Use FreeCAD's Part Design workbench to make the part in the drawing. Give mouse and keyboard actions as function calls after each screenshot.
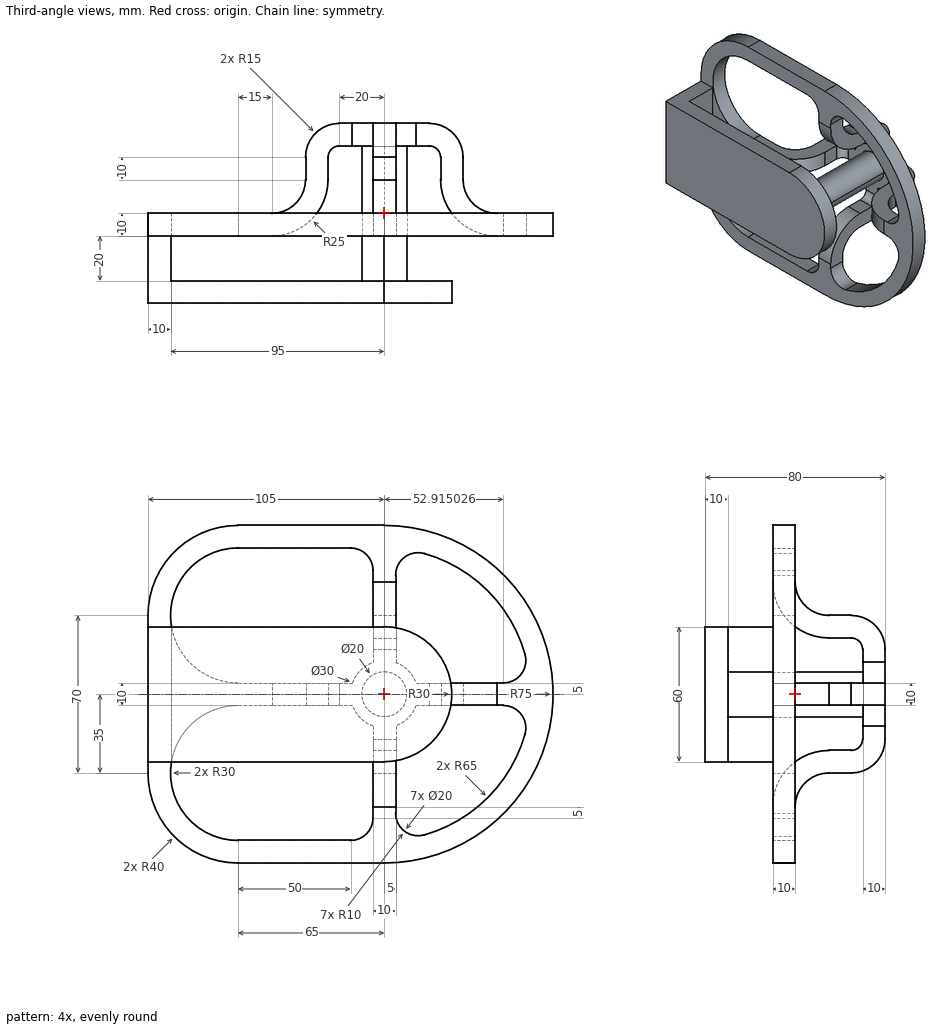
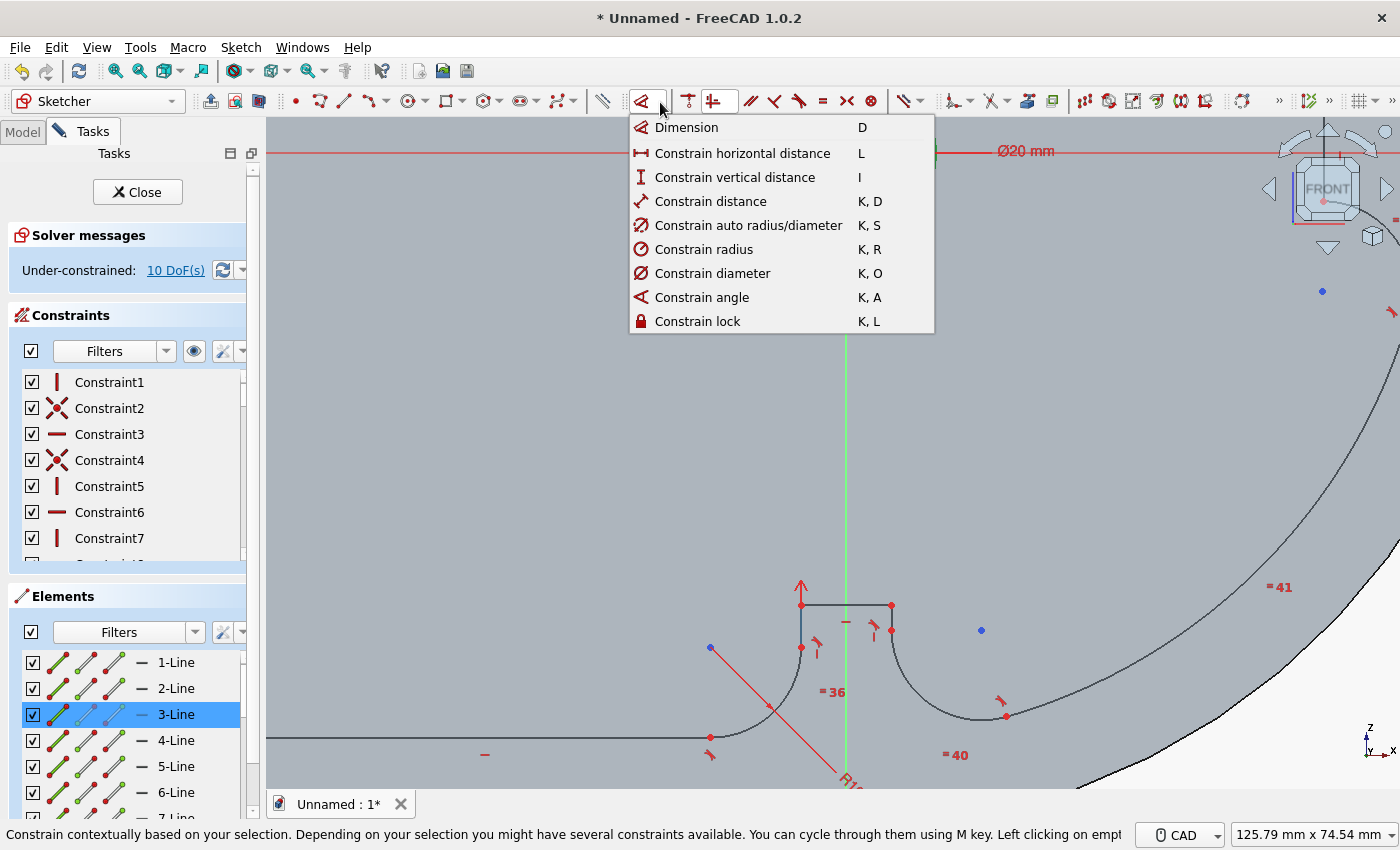
click(782, 177)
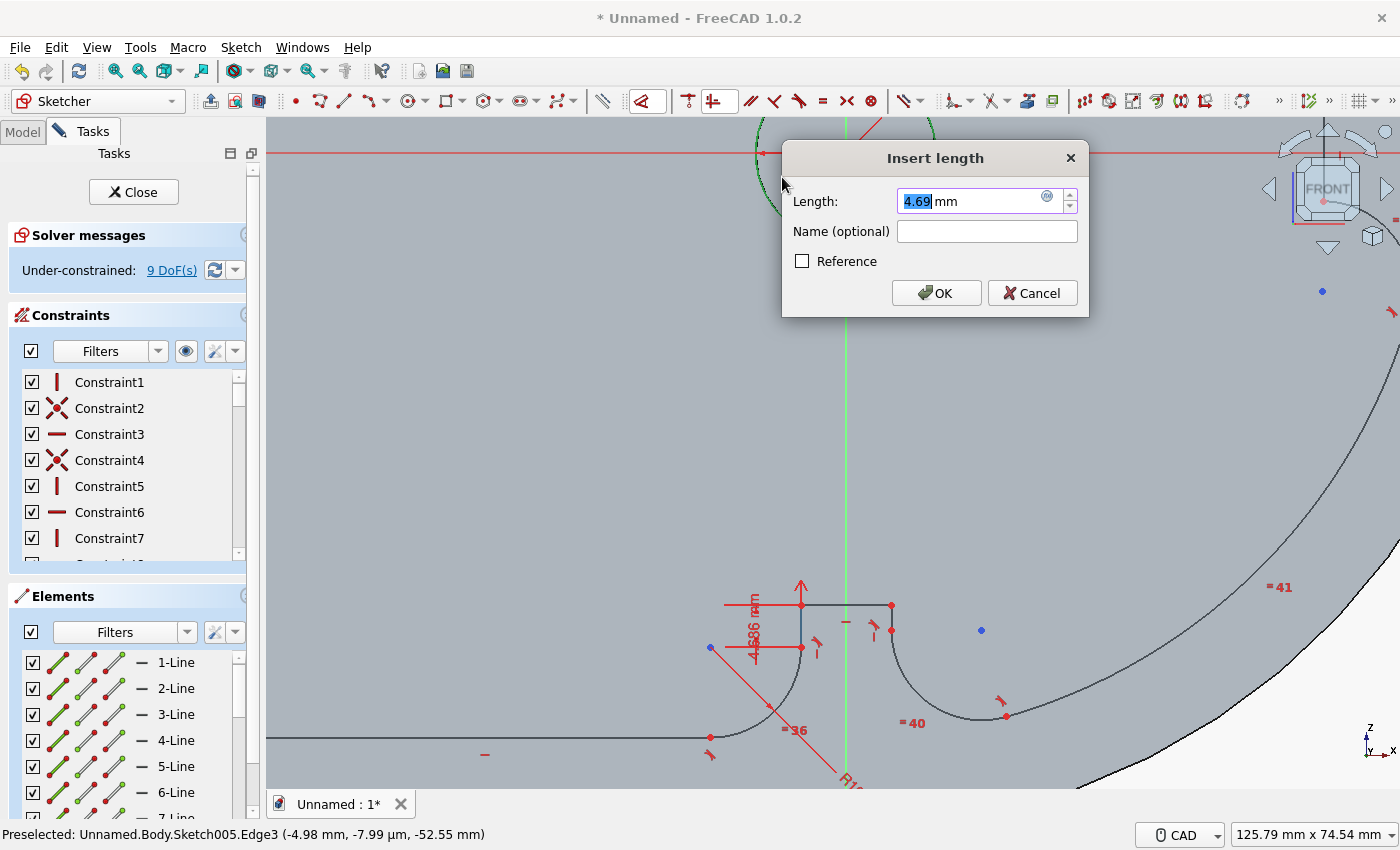
text(5)
key(Return)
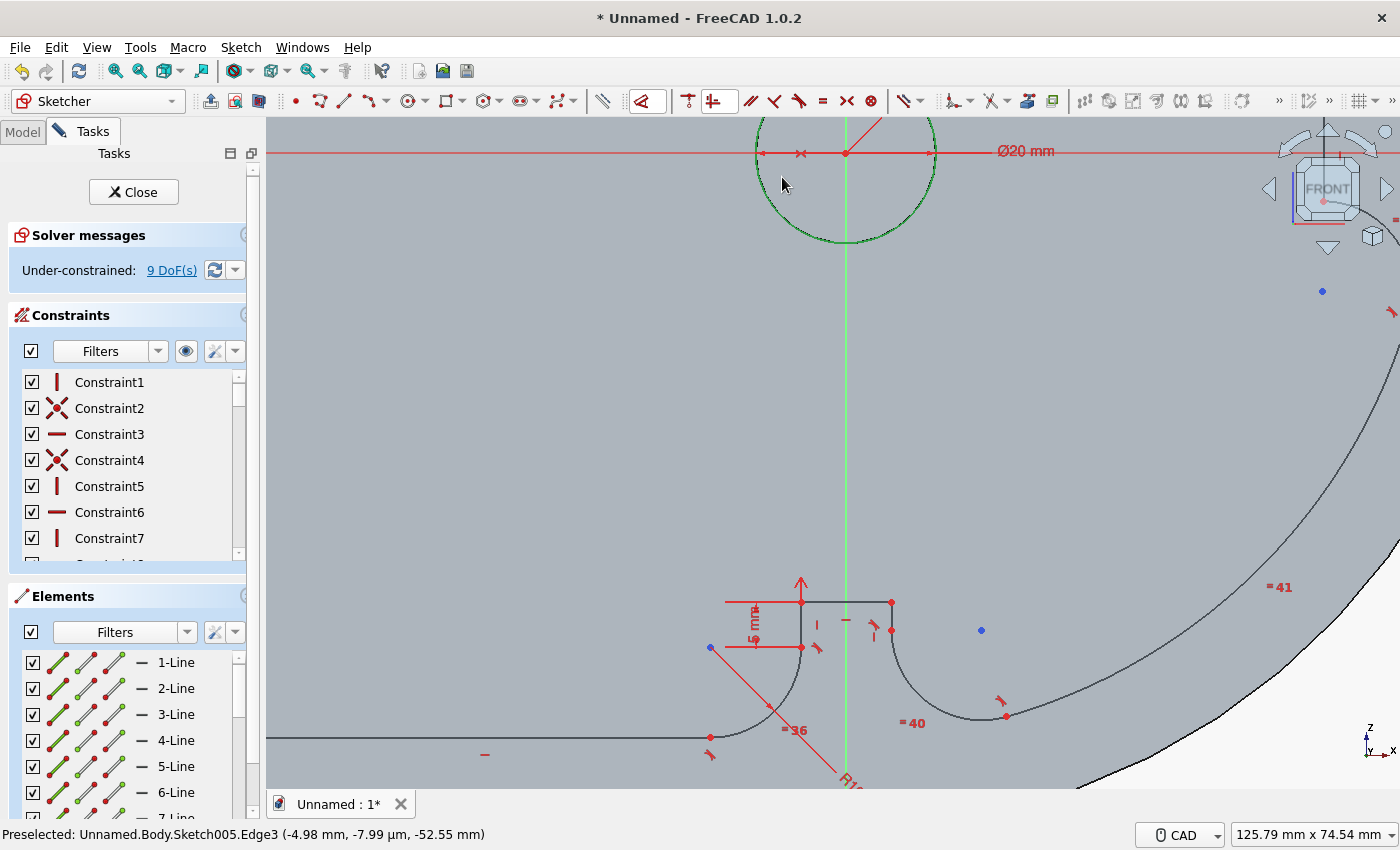
click(864, 602)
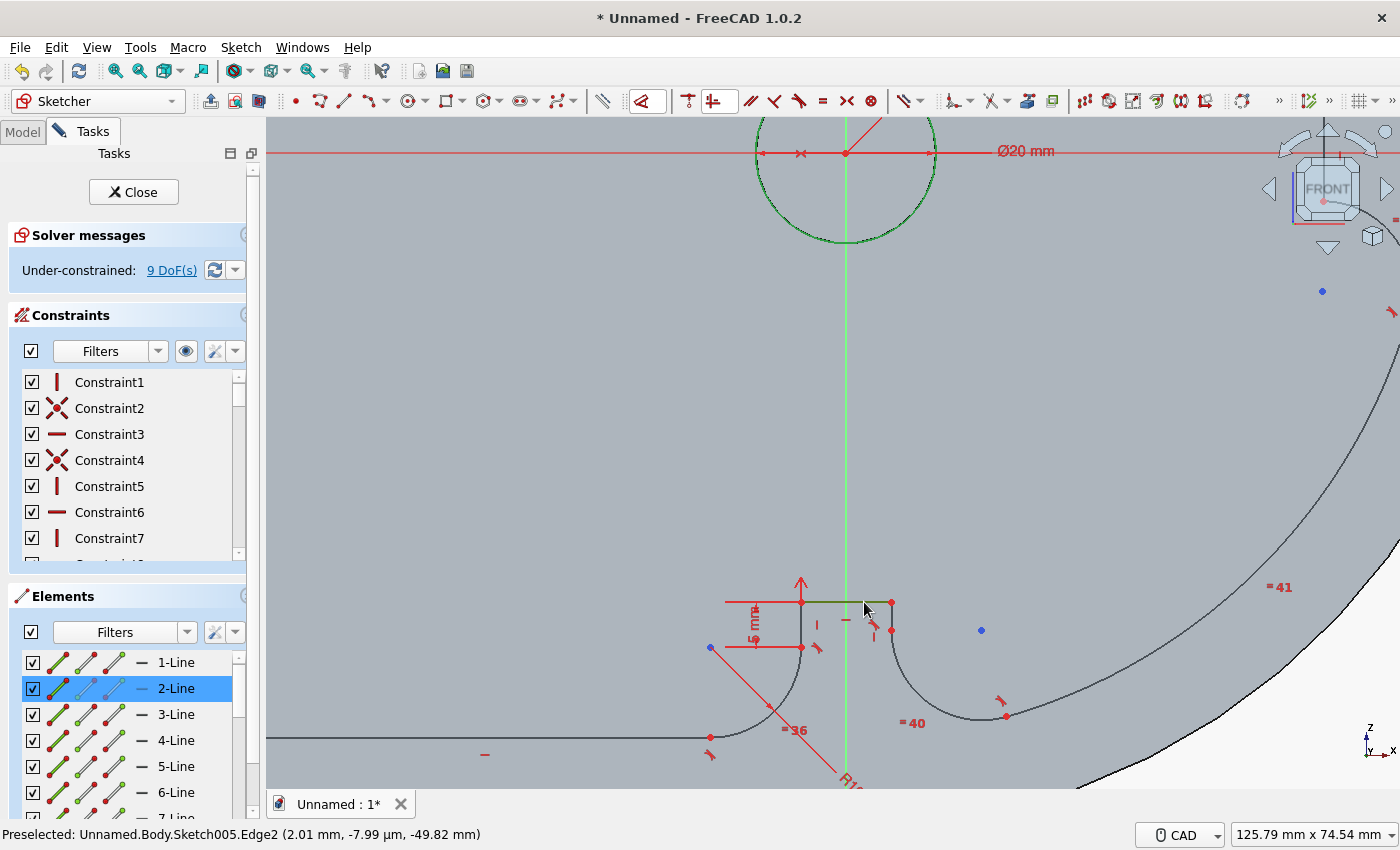
click(660, 102)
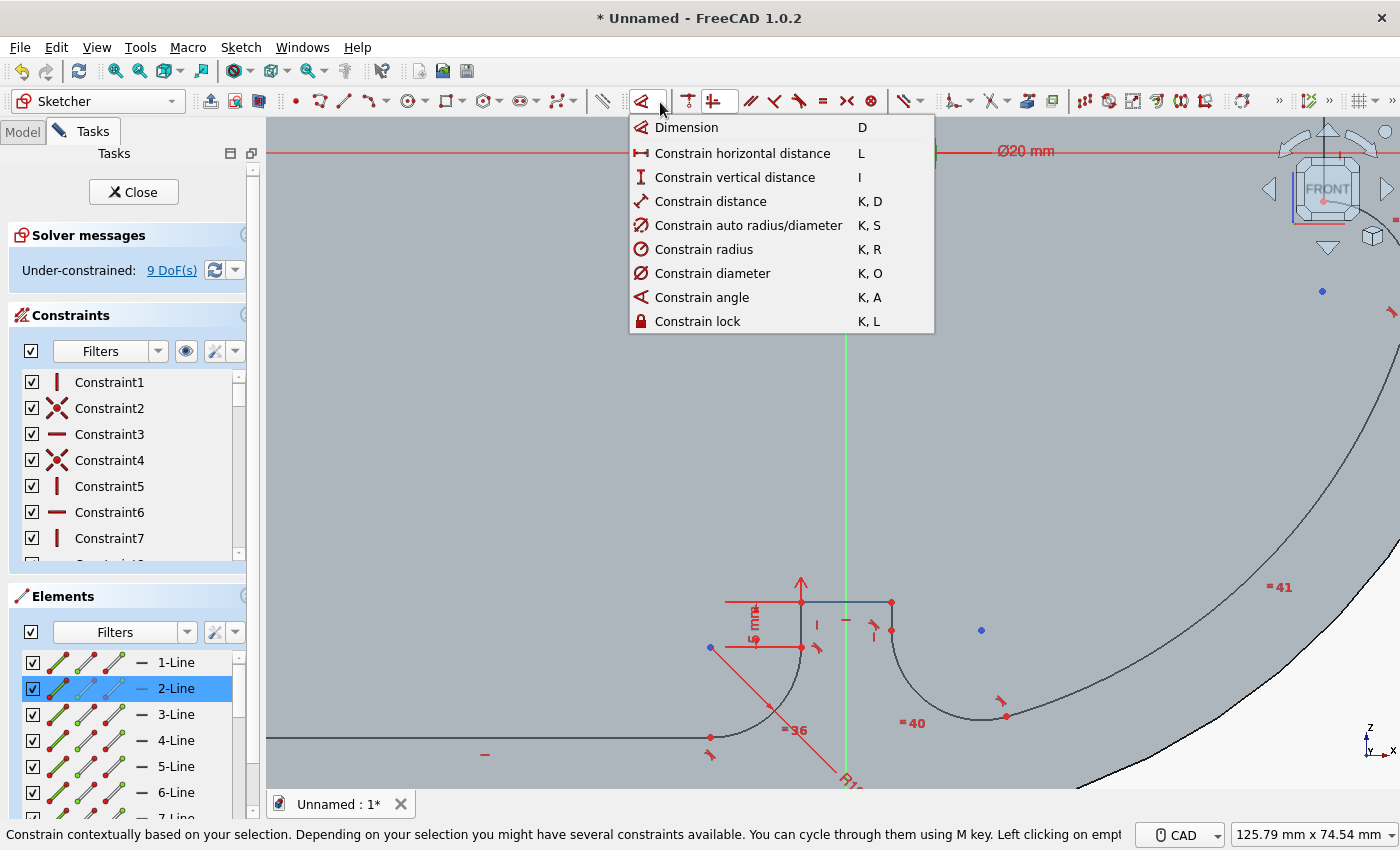
click(782, 153)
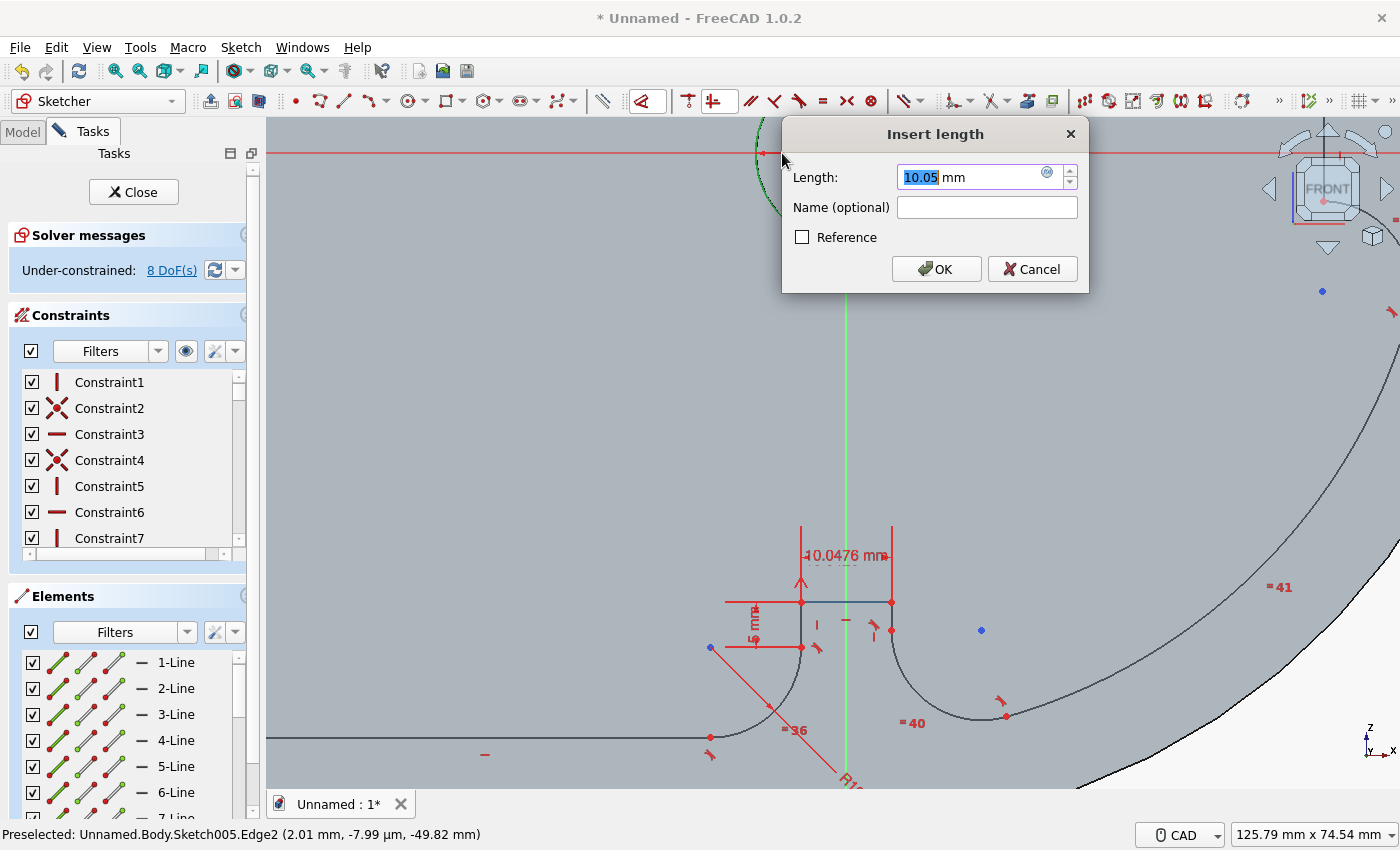
text(10)
key(Return)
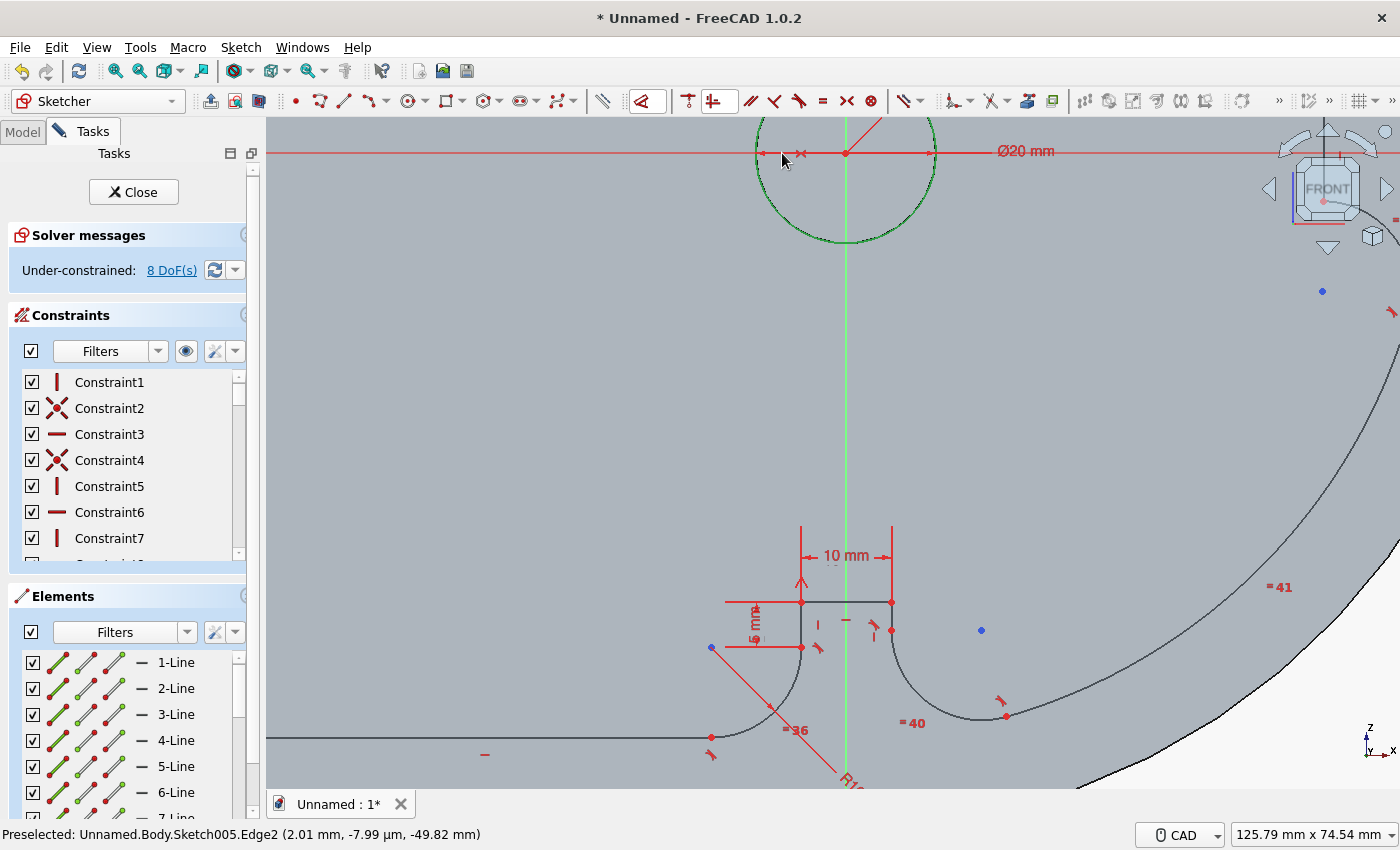
click(576, 738)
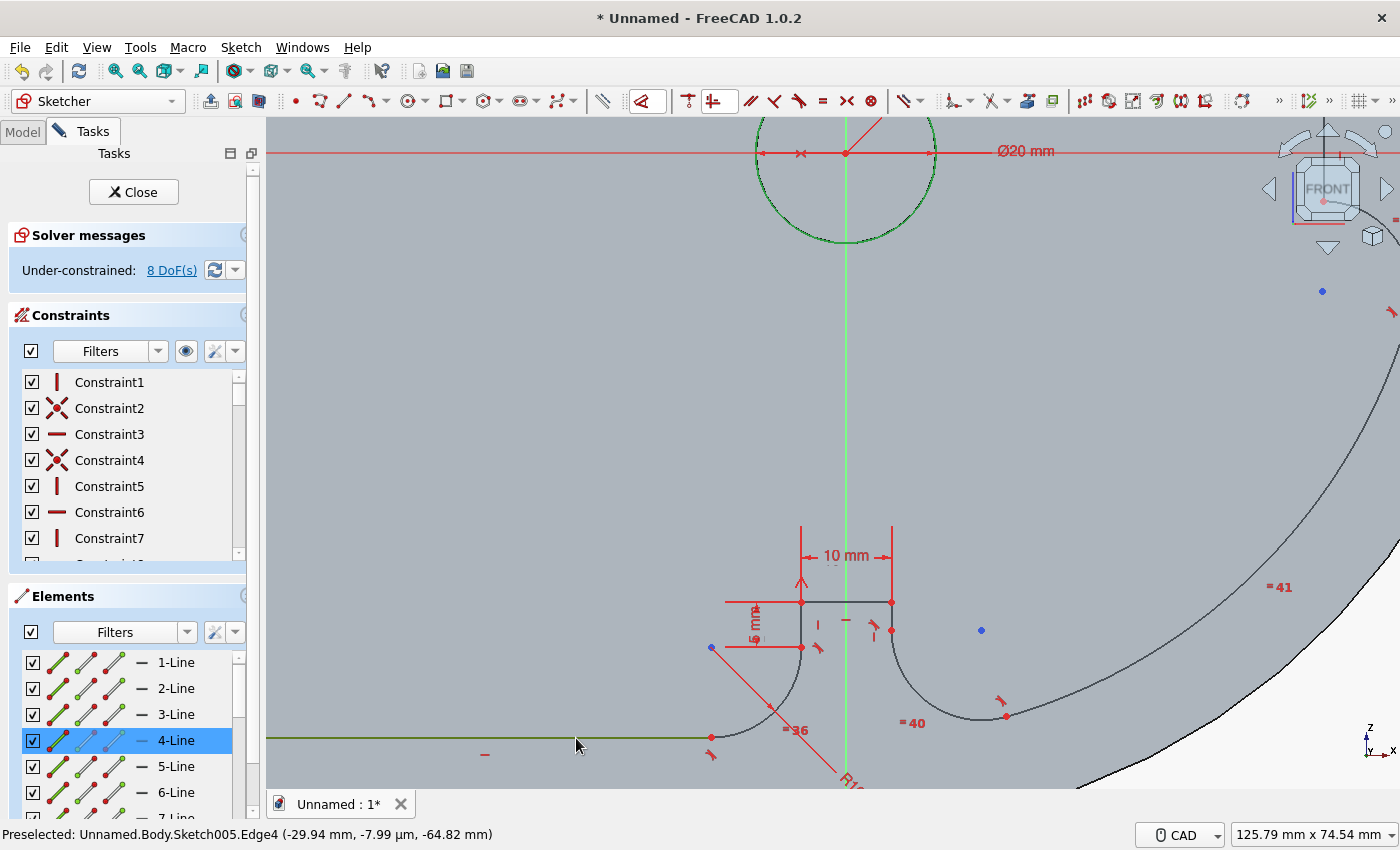
key(l)